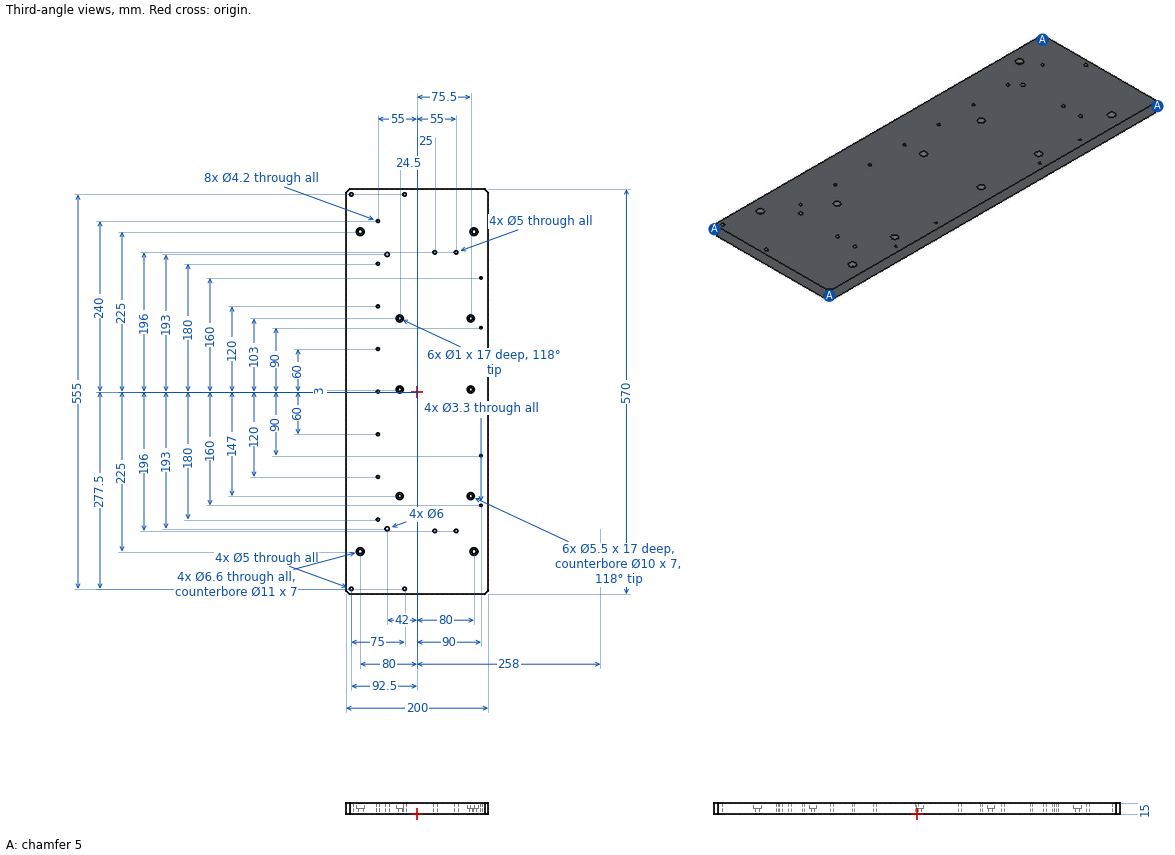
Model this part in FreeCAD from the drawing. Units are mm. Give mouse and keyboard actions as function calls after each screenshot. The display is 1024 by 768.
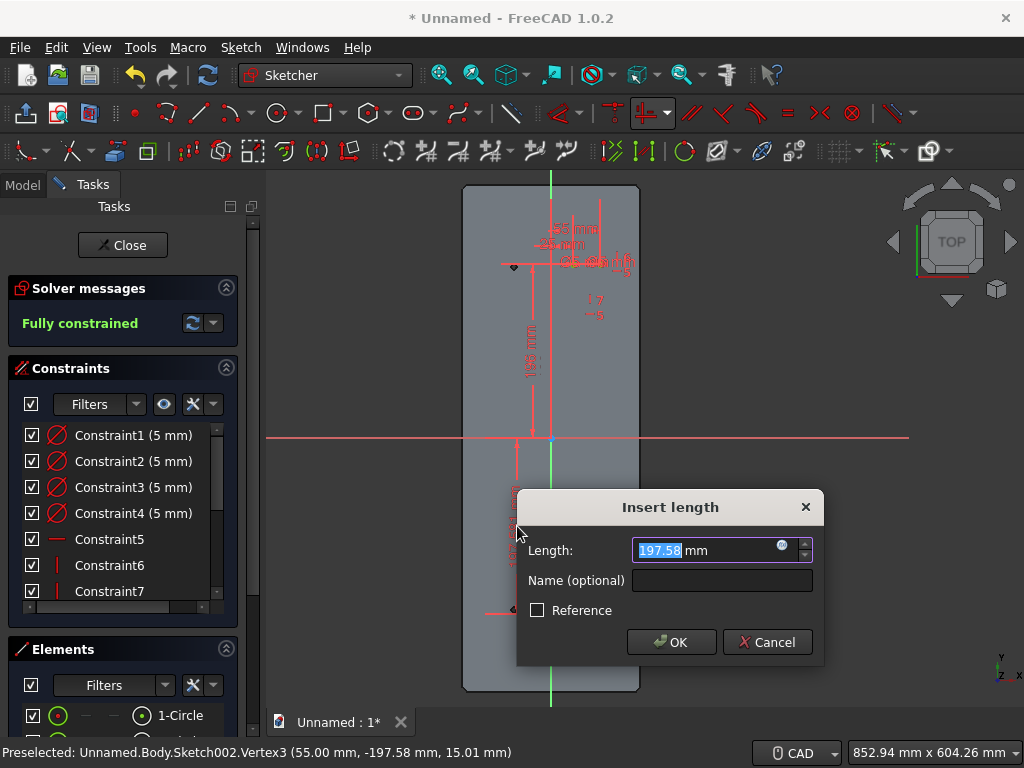
text(196)
key(Return)
key(Escape)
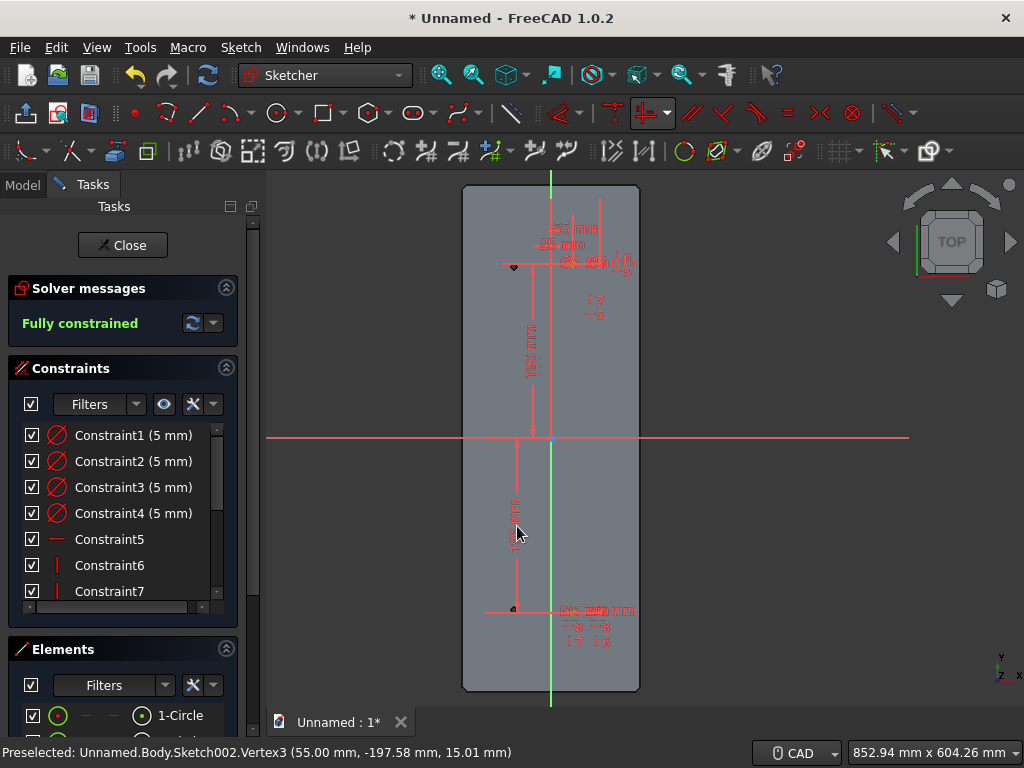
click(123, 245)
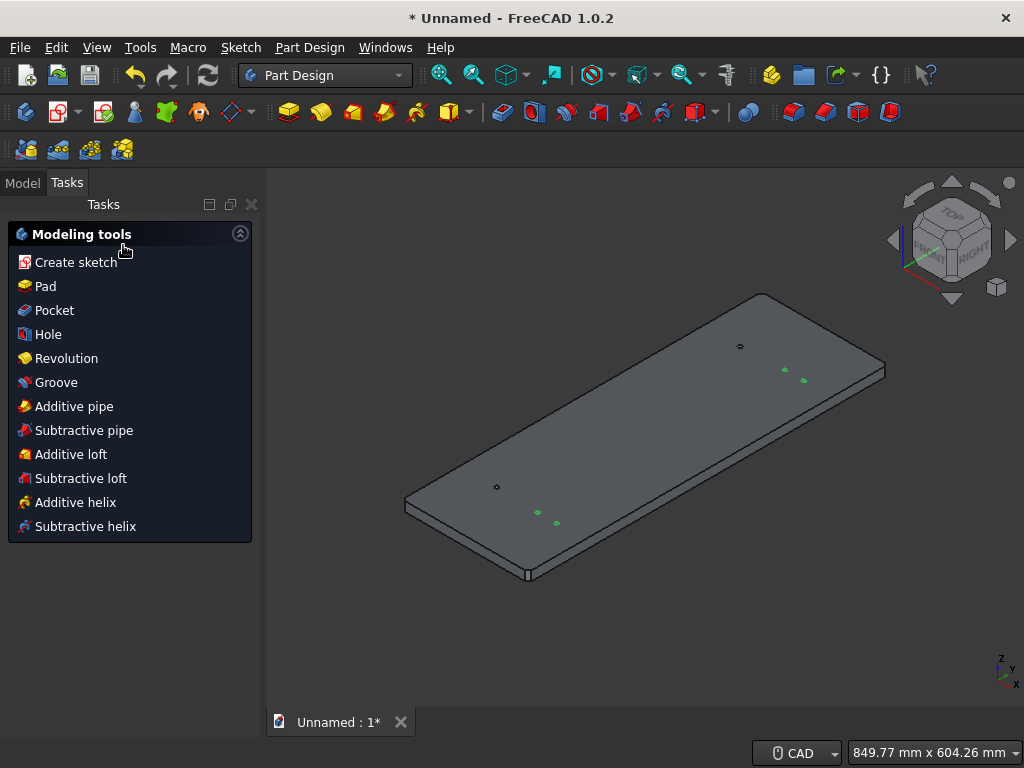
click(536, 112)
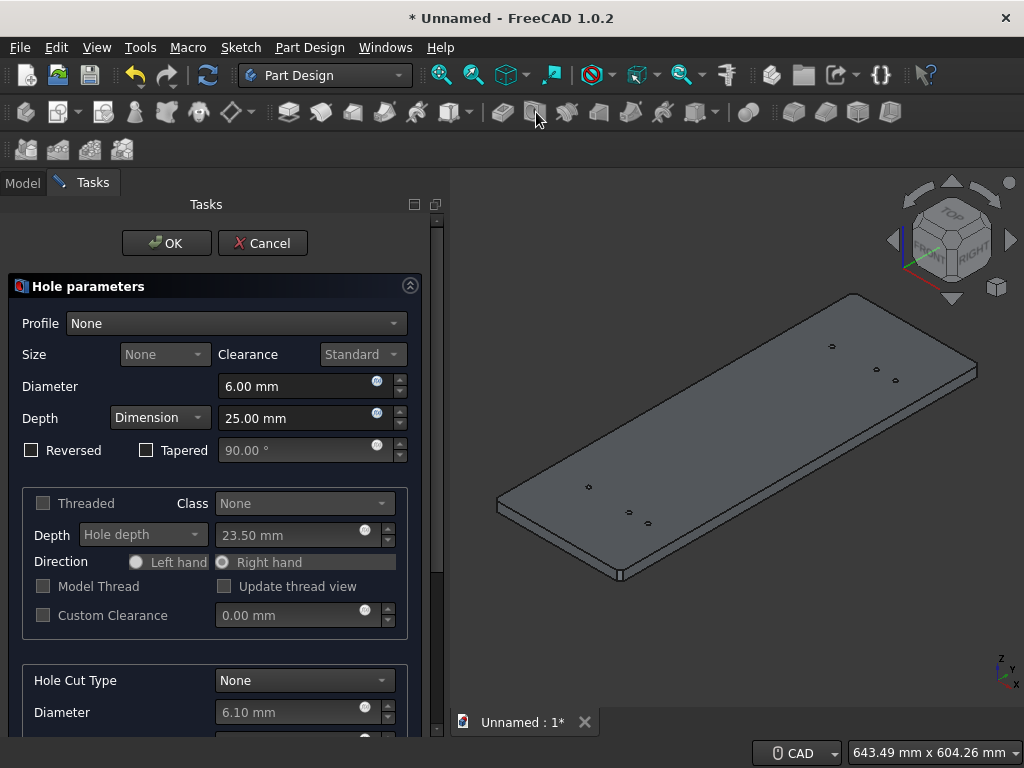
triple_click(305, 386)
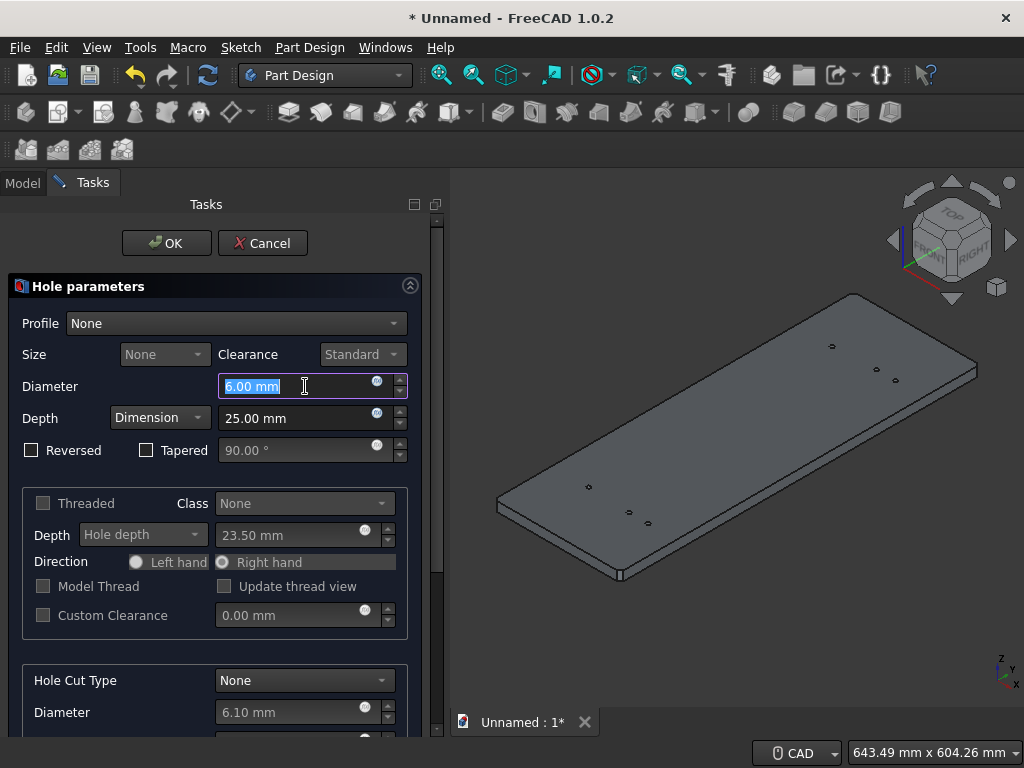
text(5)
key(Tab)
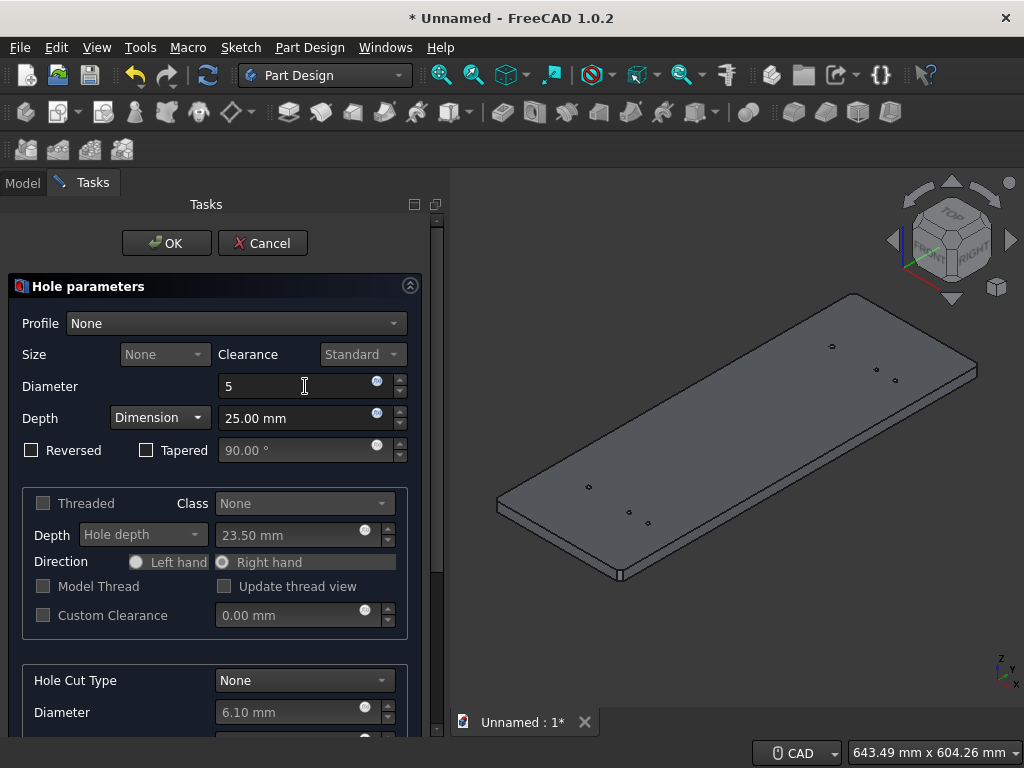
click(161, 418)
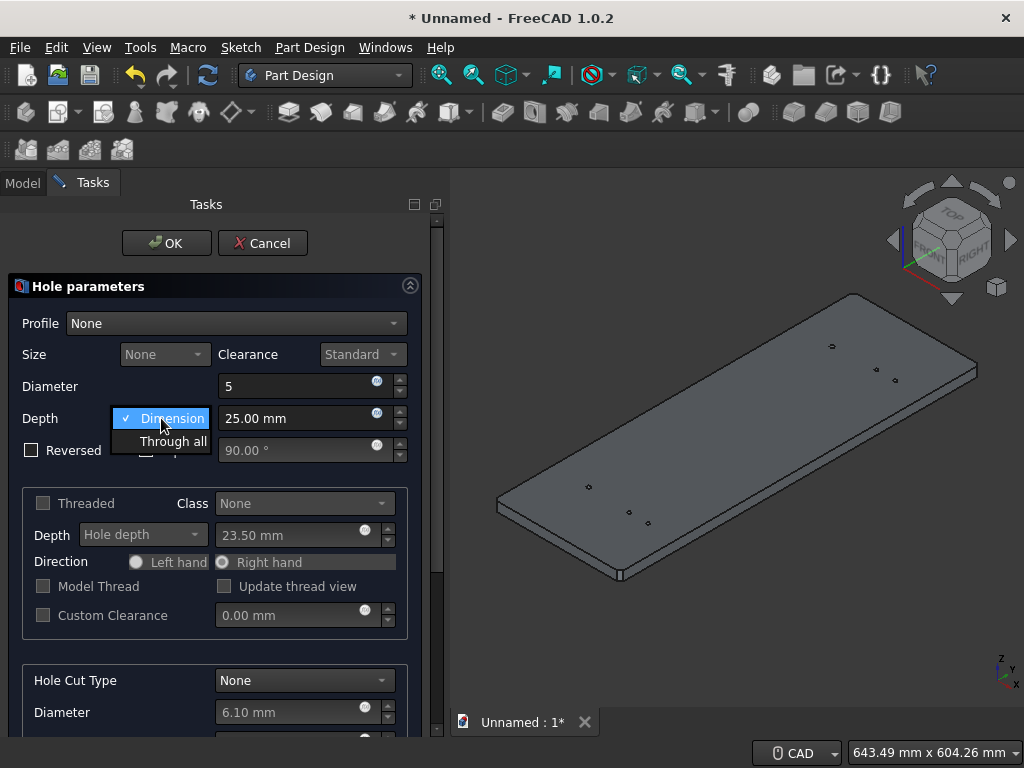
click(160, 442)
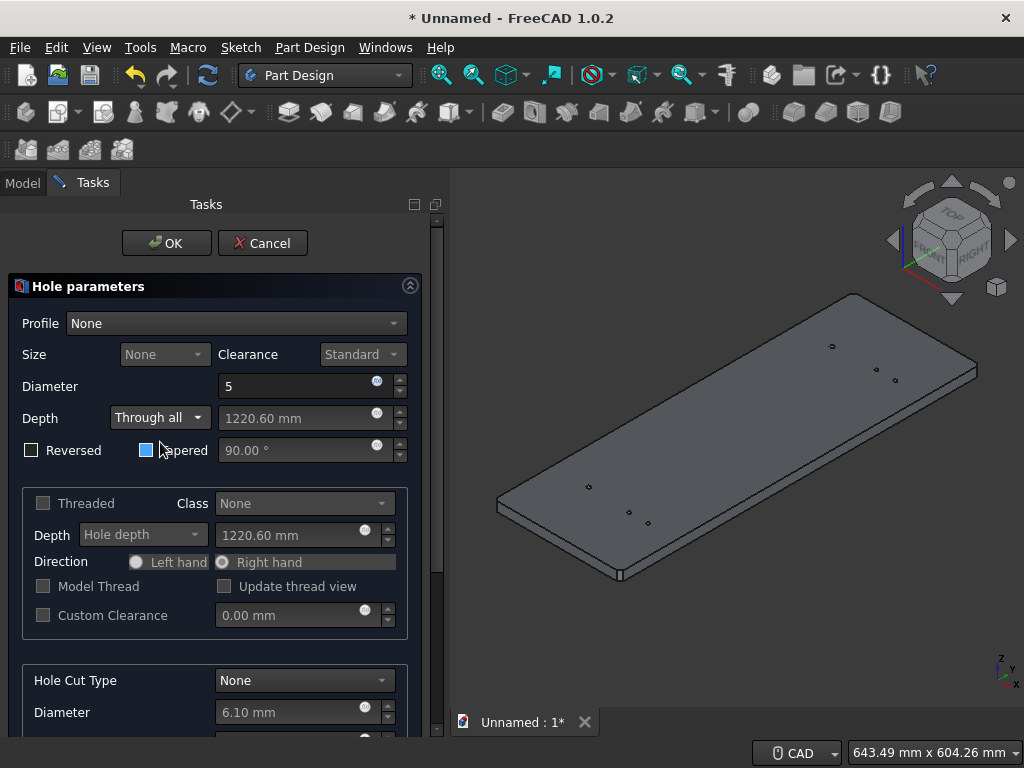
click(167, 243)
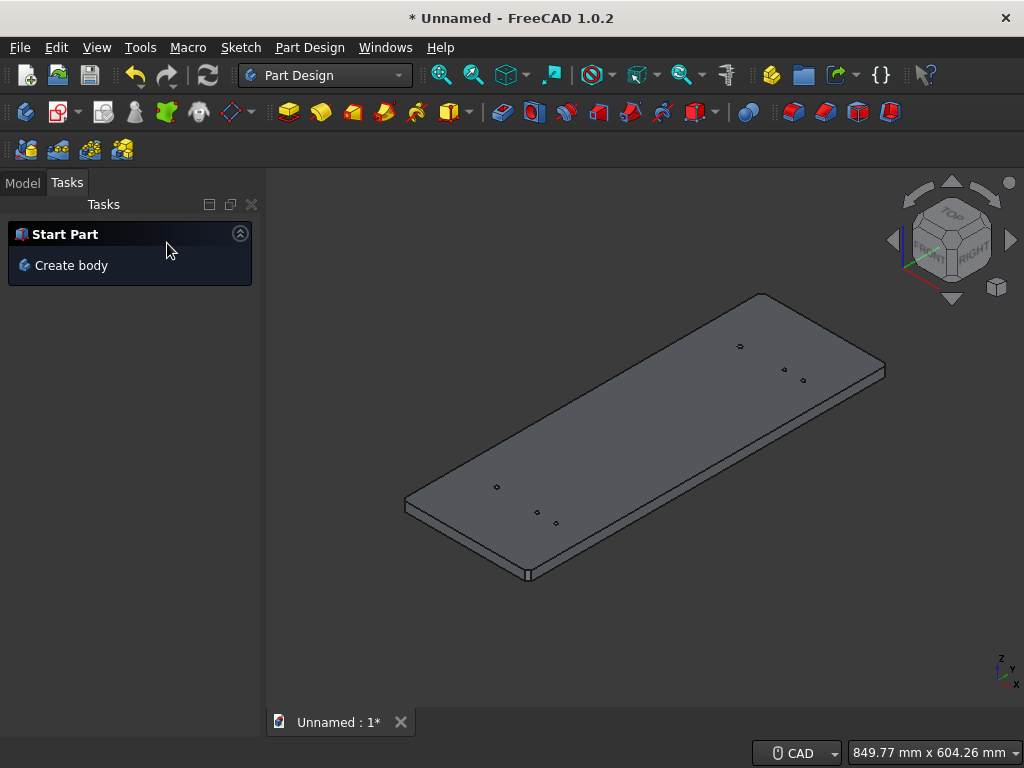
click(696, 401)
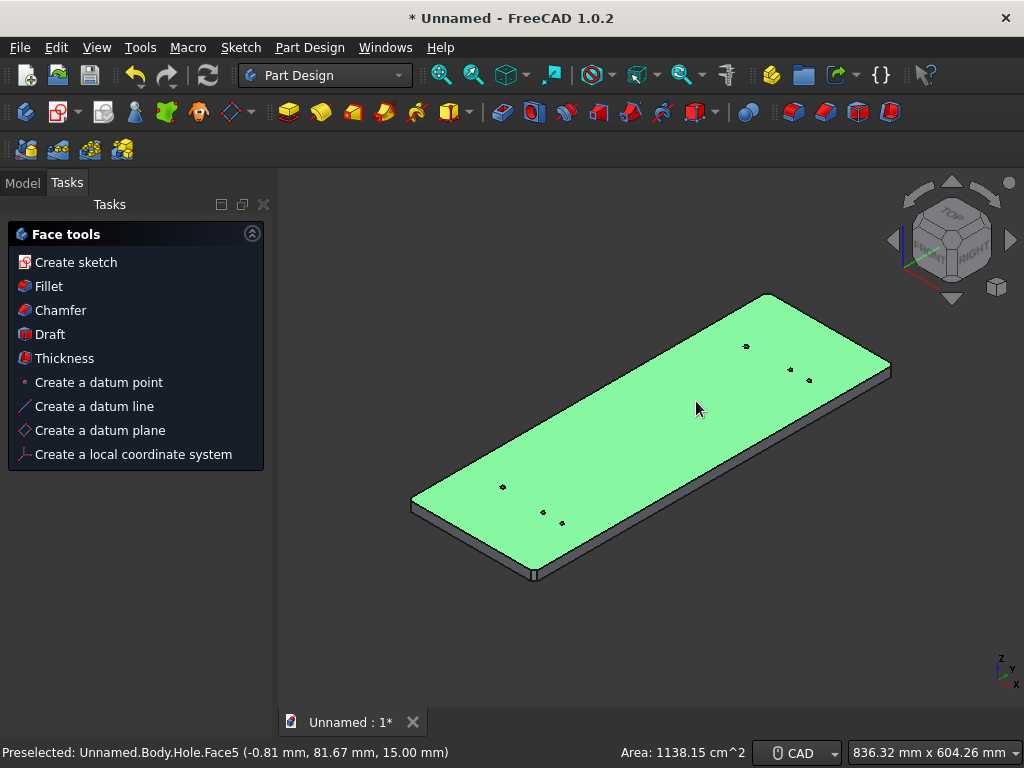
click(58, 112)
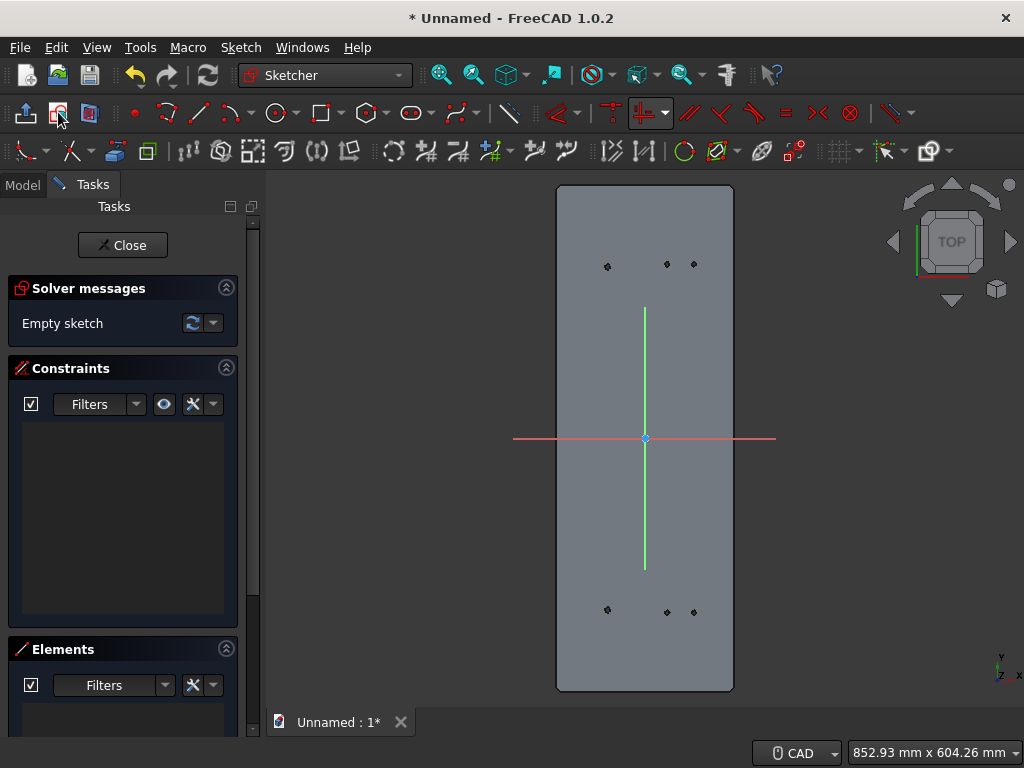
click(276, 114)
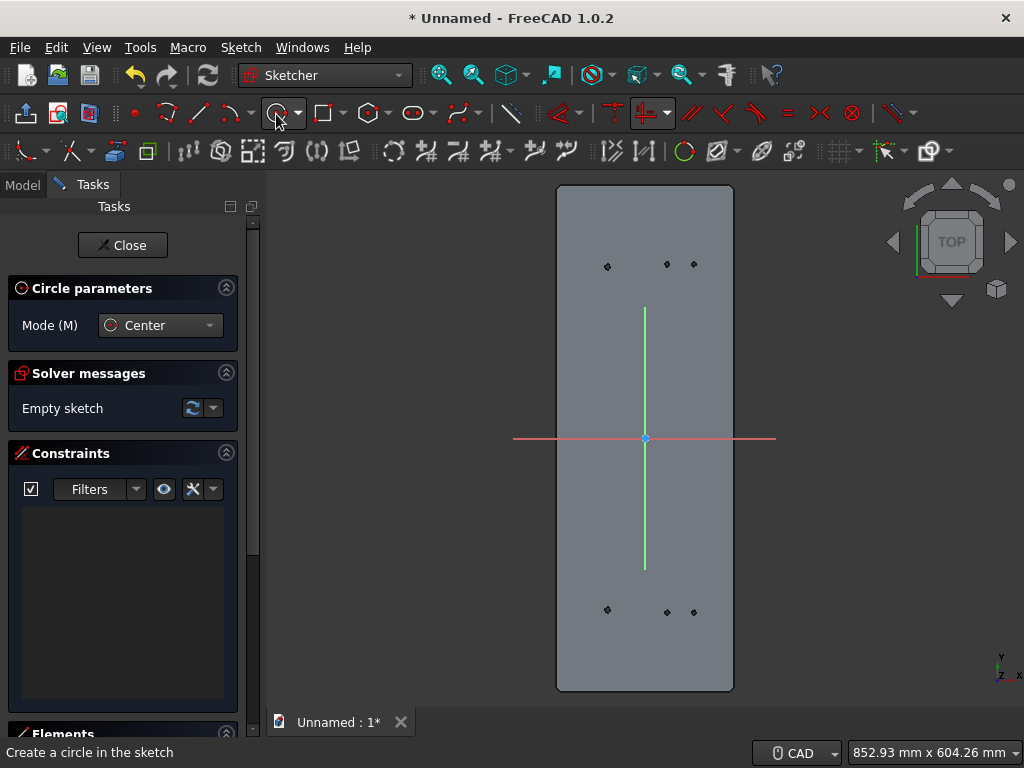
scroll(596, 225, up, 13)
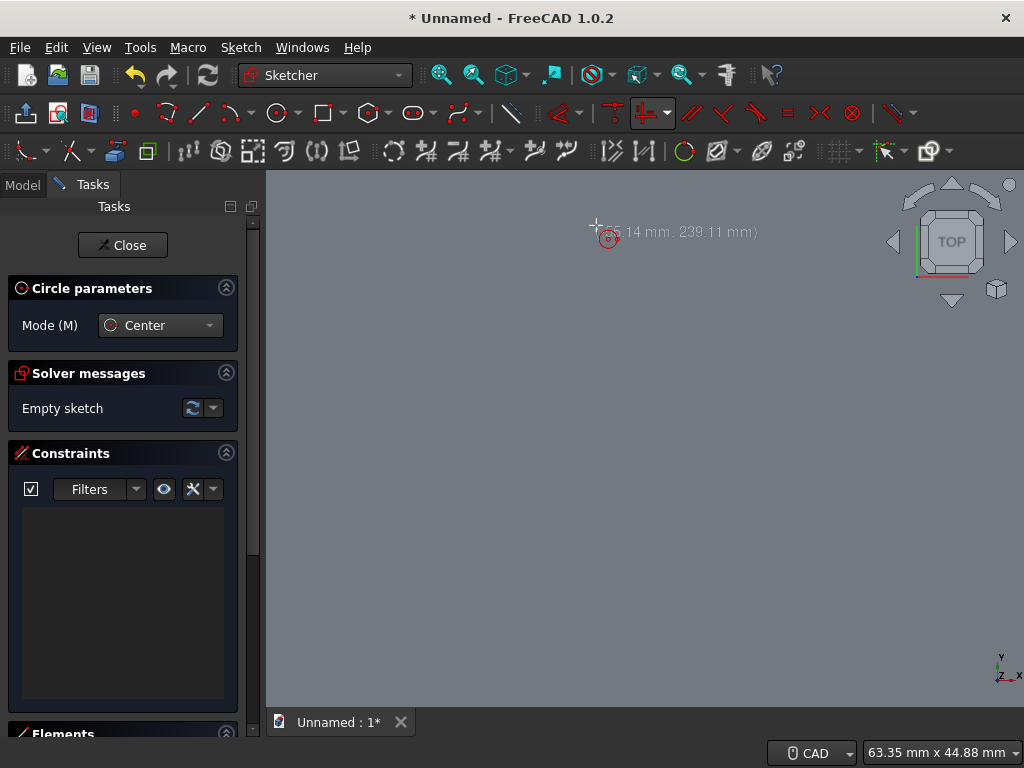
scroll(555, 290, down, 14)